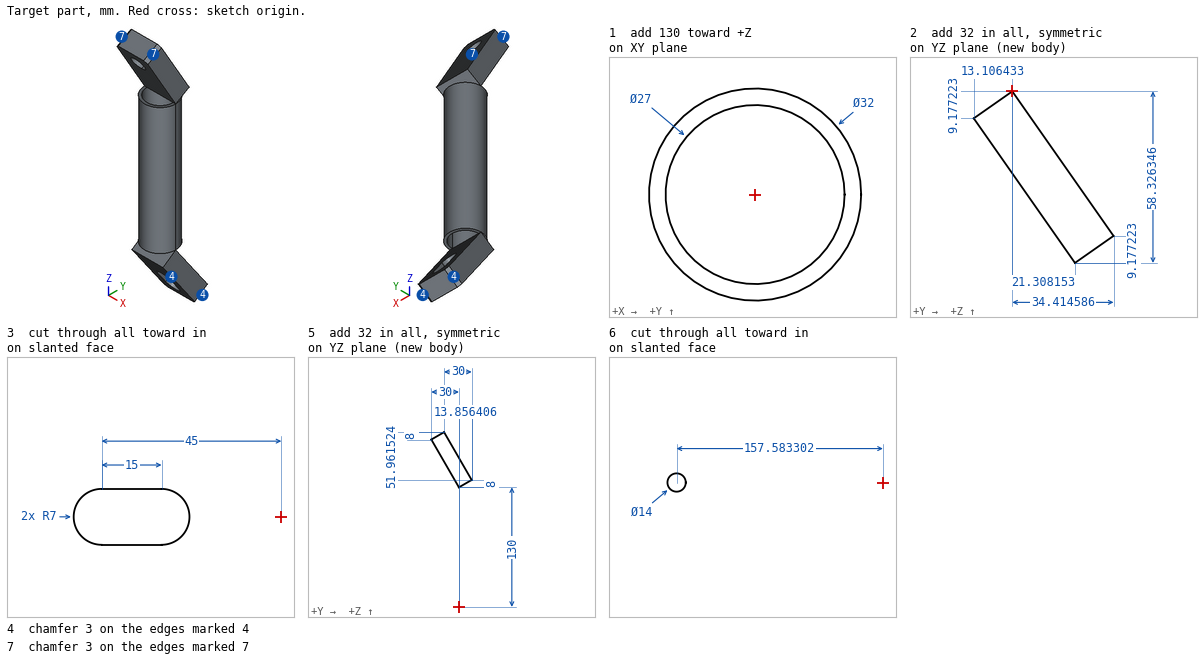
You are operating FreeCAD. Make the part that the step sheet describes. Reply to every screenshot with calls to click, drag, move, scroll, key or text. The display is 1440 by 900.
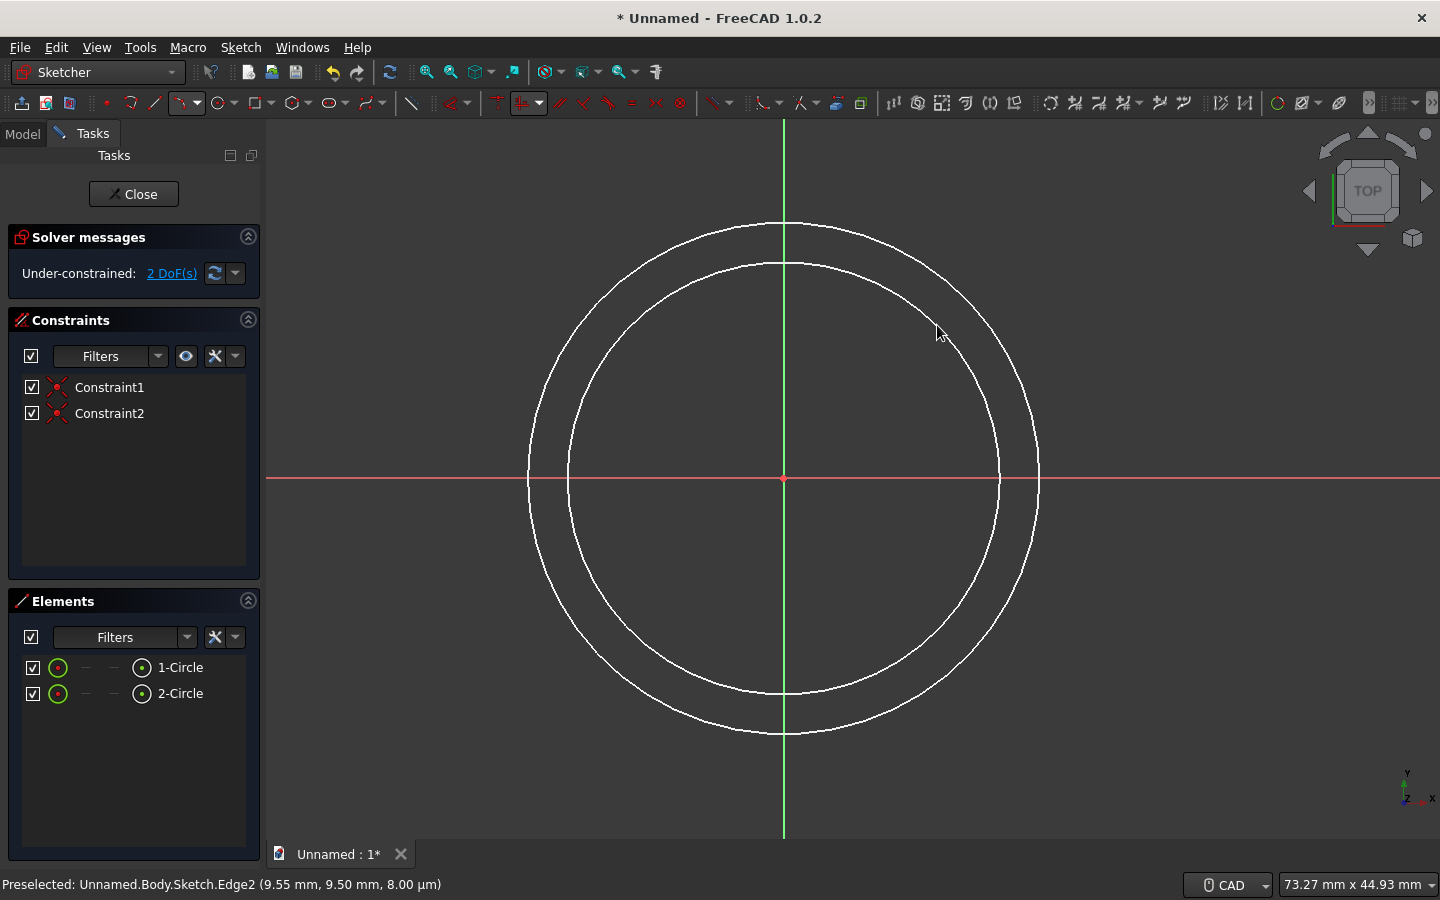
key(d)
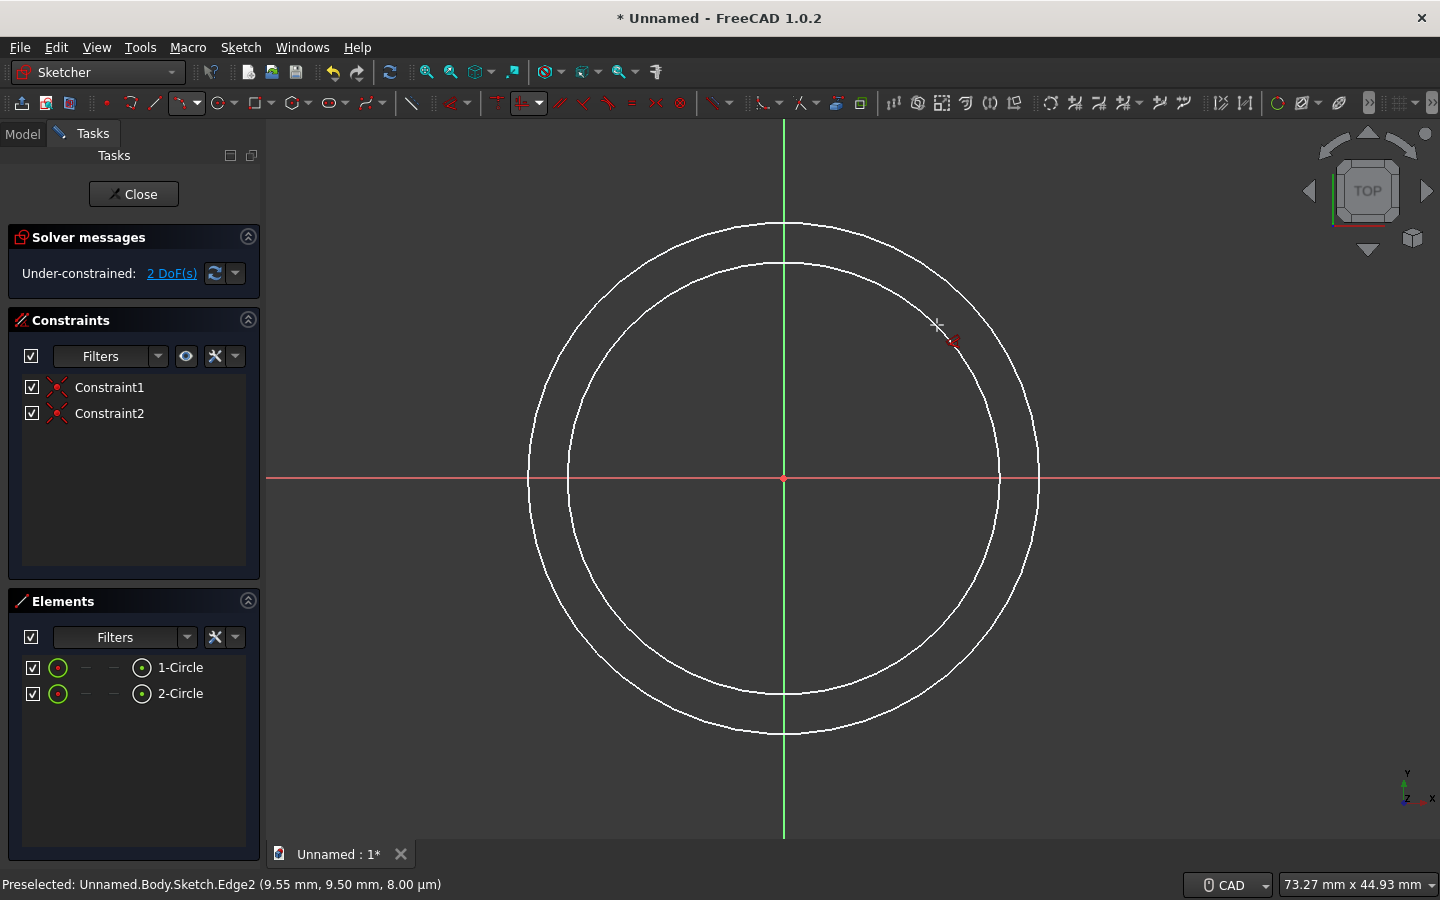
click(964, 297)
click(987, 274)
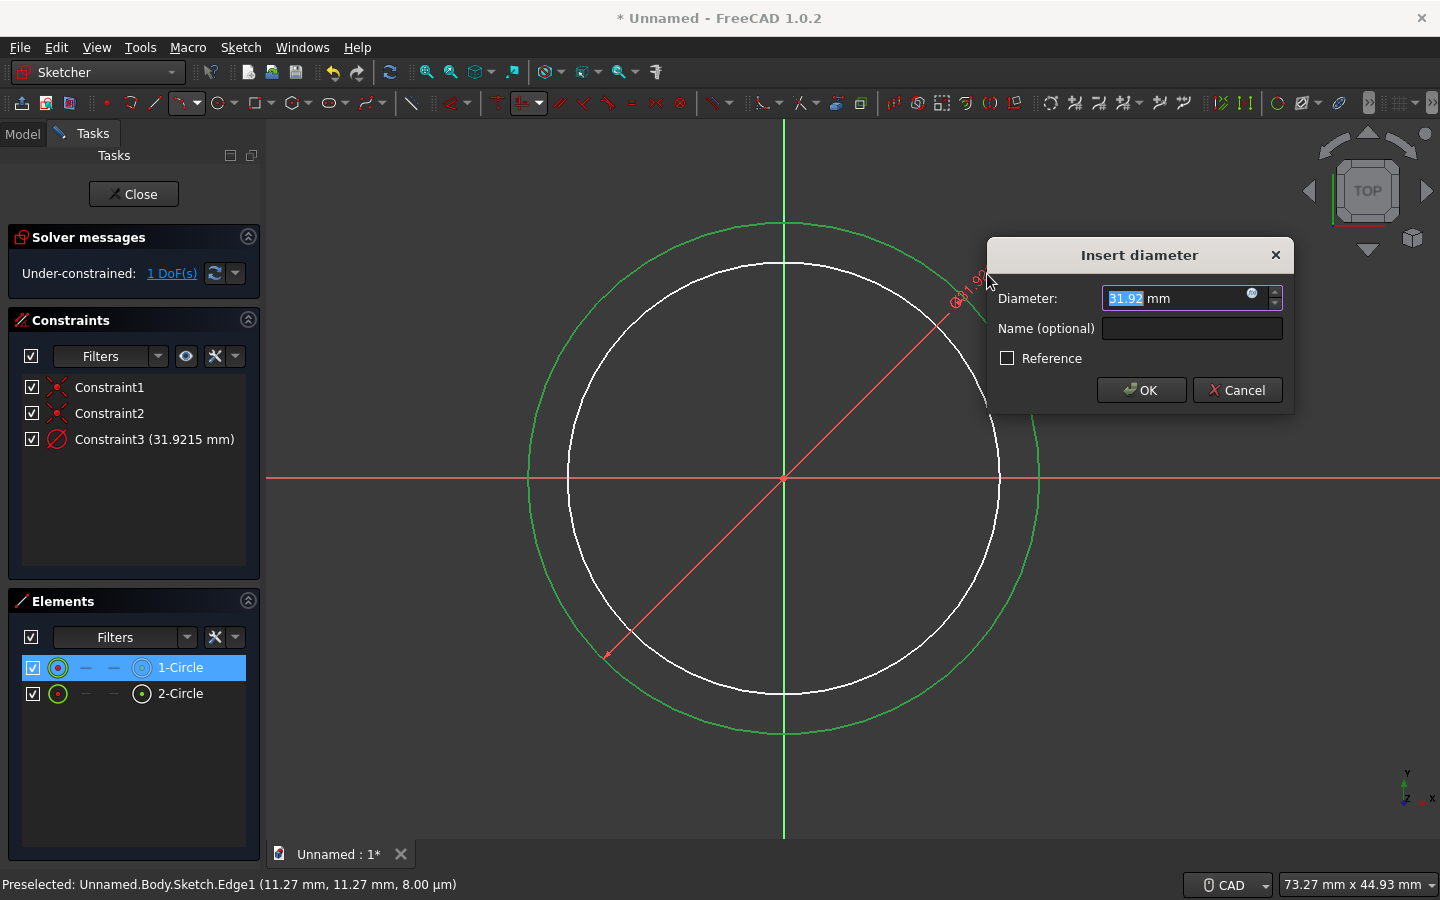
text(32)
key(Return)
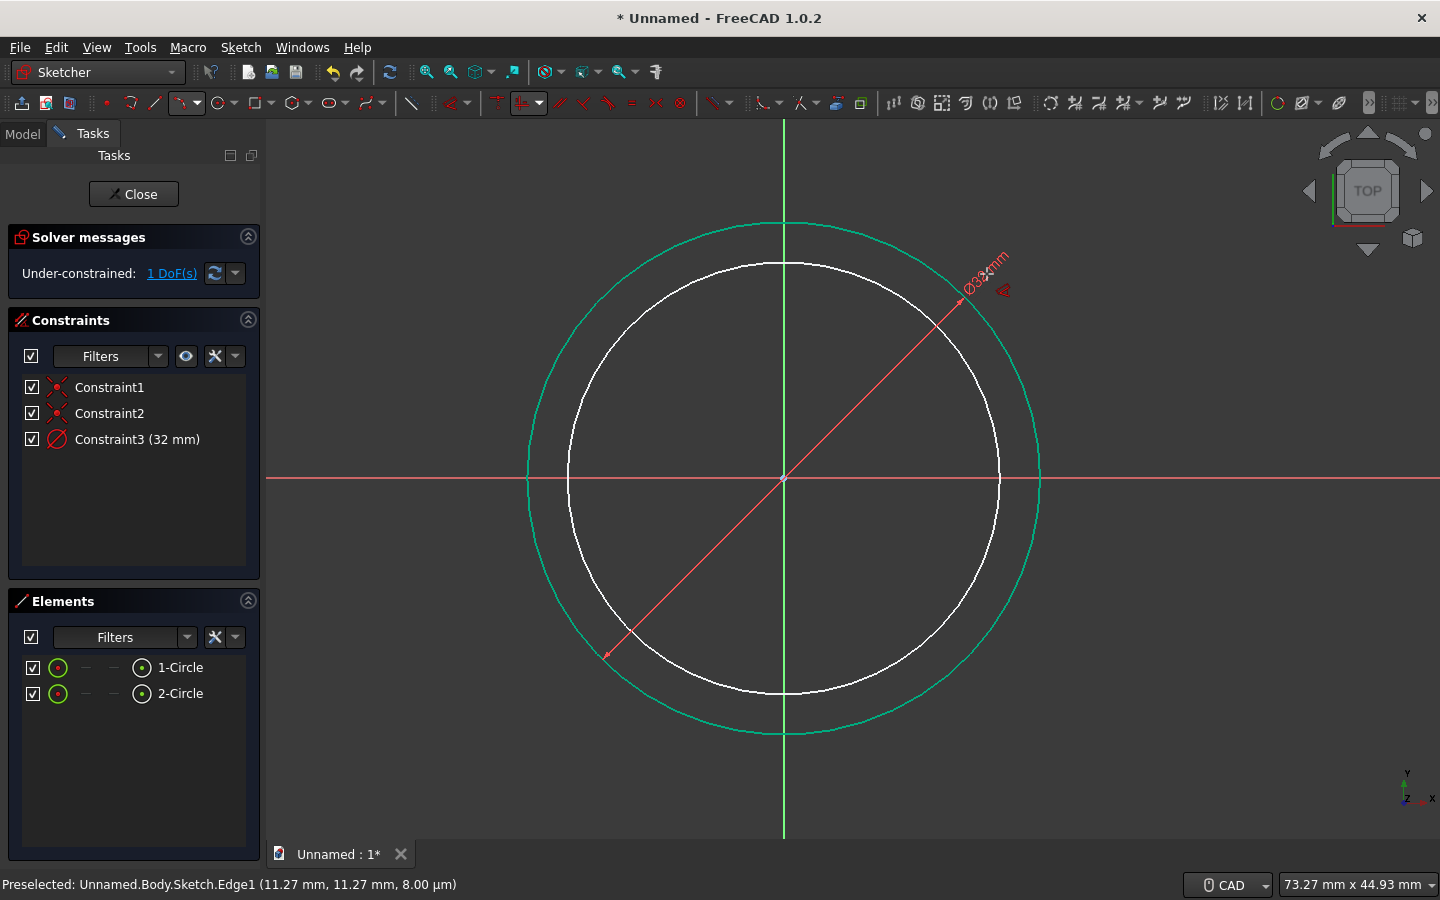
click(936, 325)
click(1044, 401)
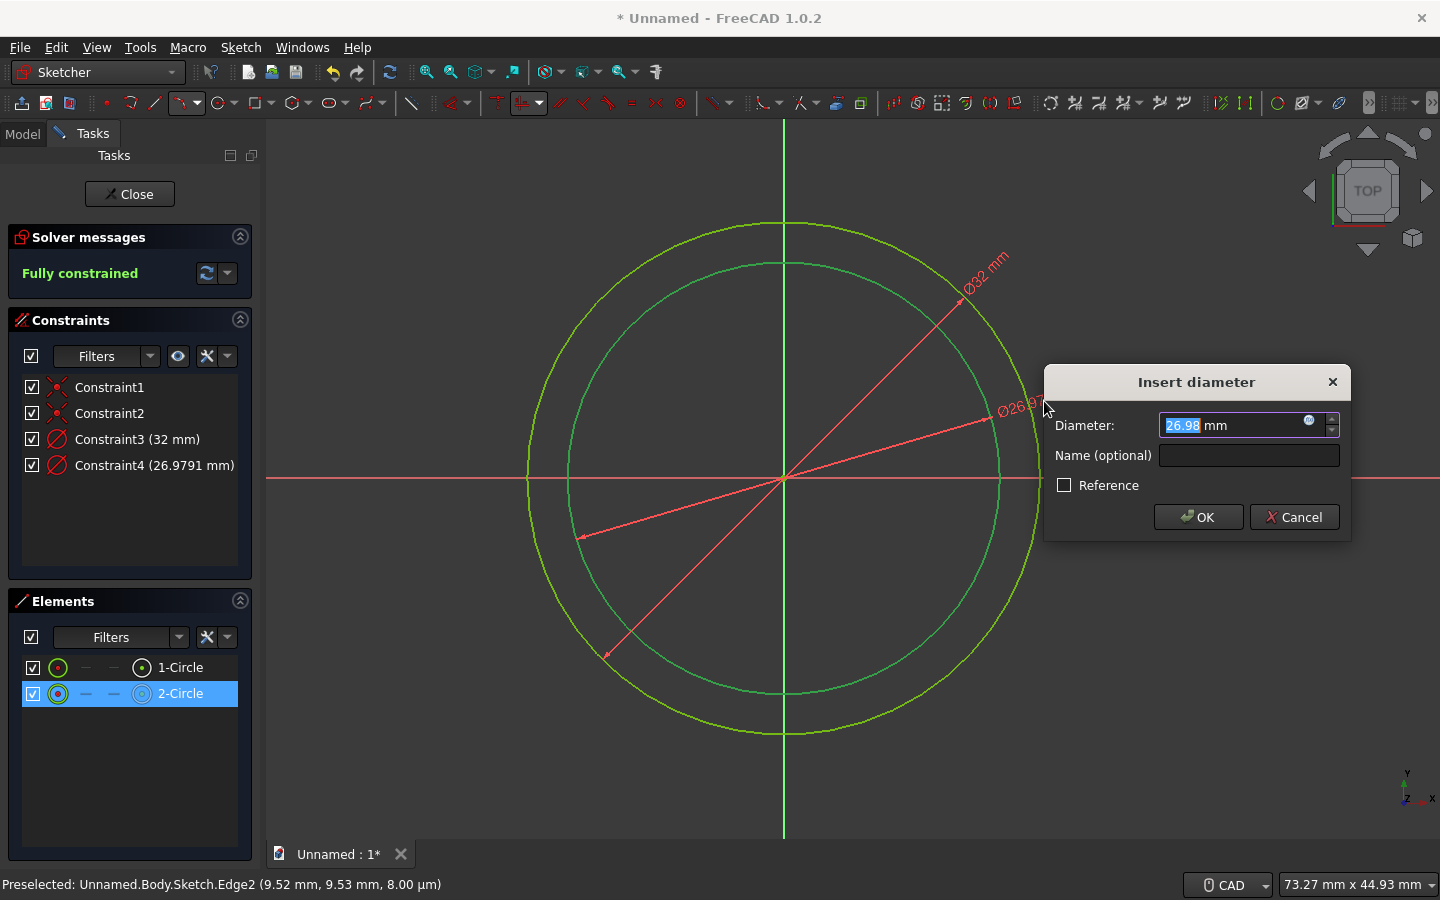
text(27)
key(Return)
key(Escape)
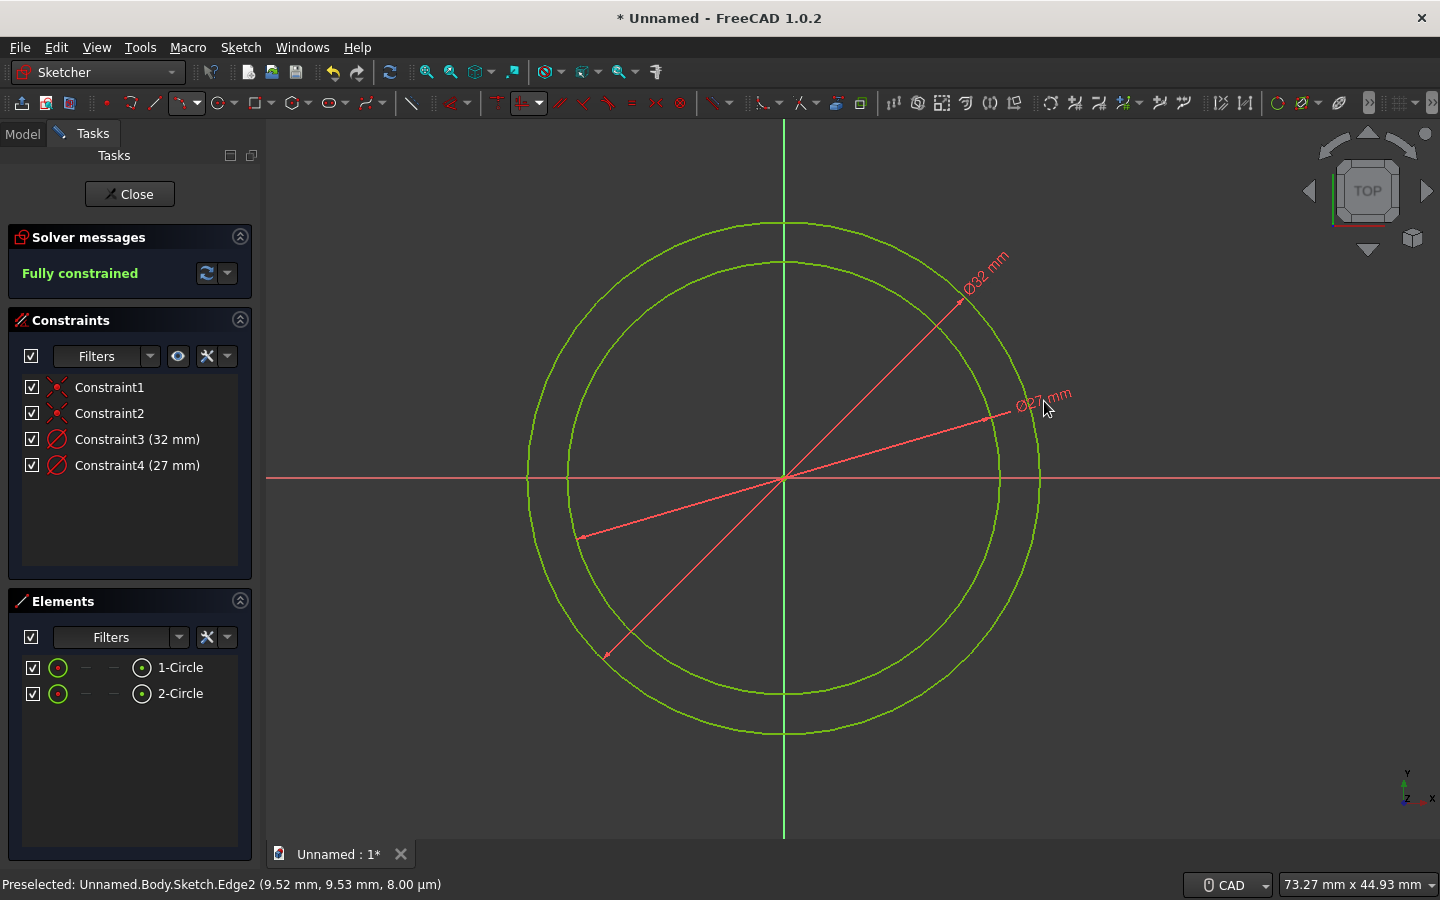
click(130, 194)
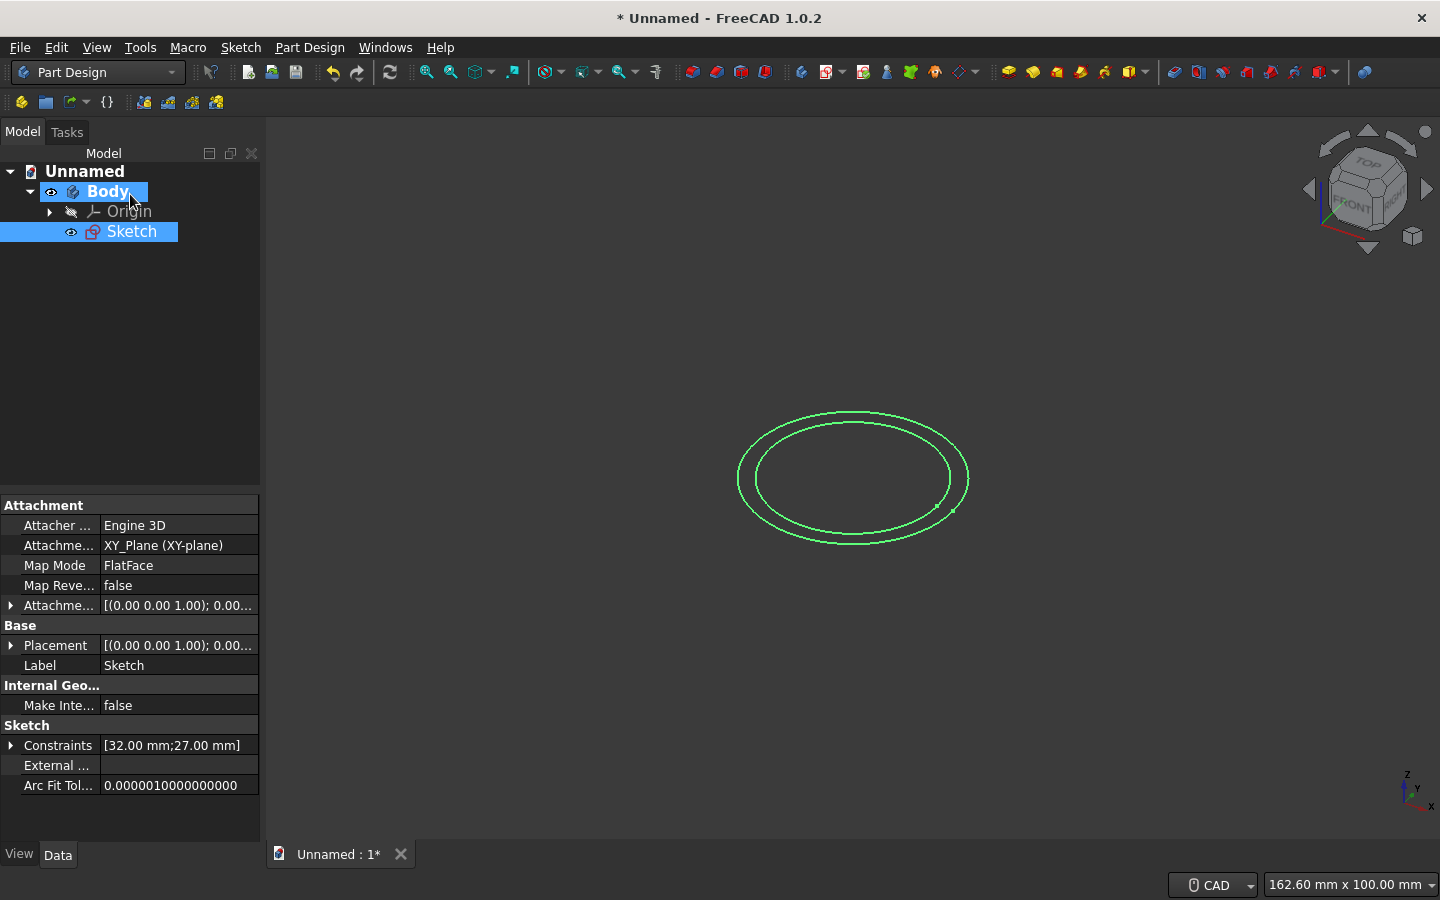
click(1010, 72)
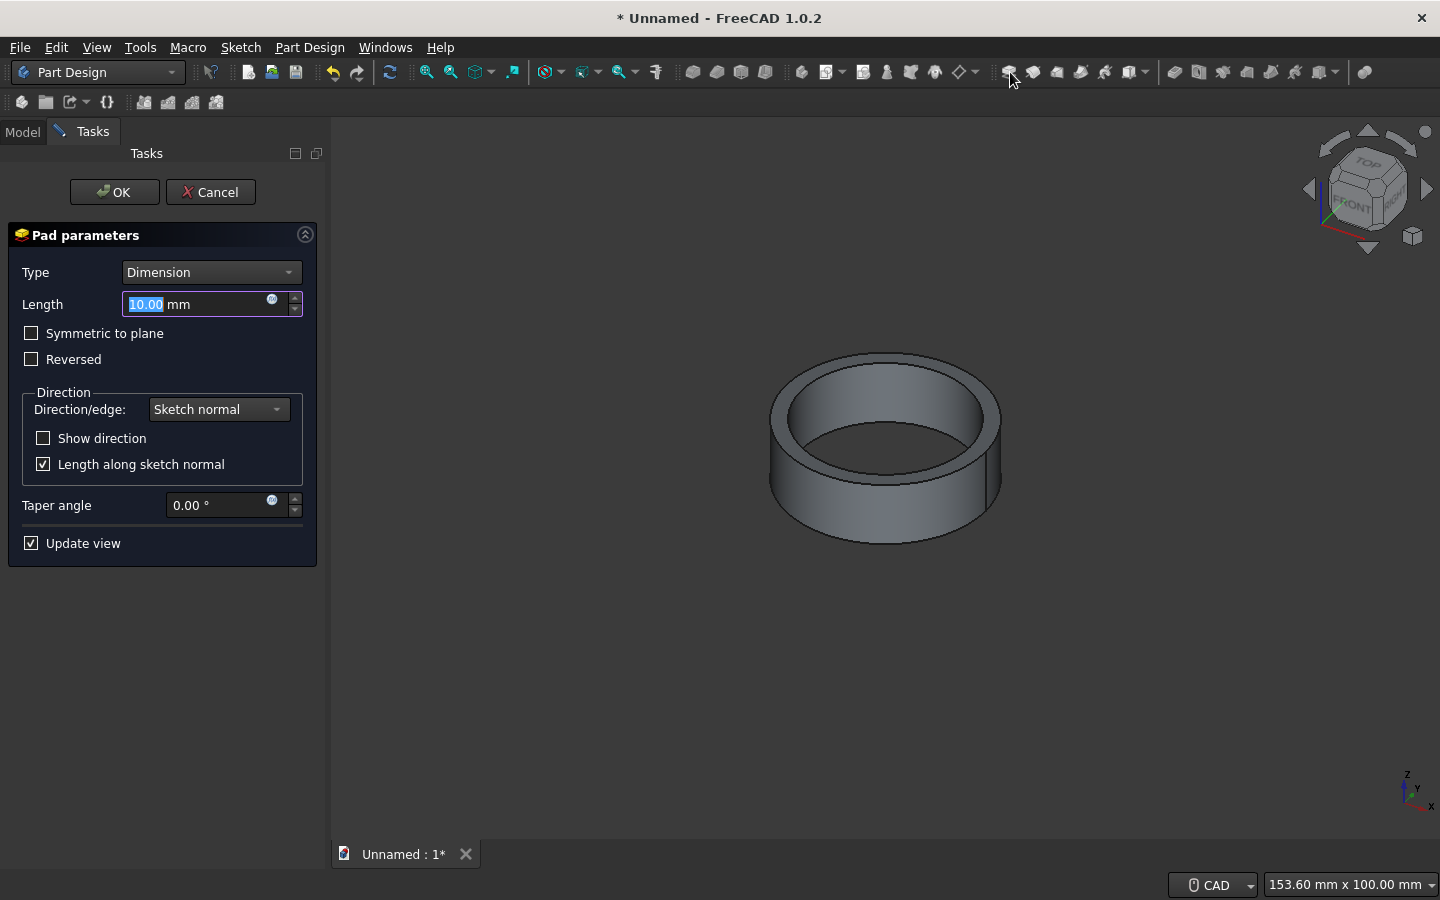
text(130)
key(Tab)